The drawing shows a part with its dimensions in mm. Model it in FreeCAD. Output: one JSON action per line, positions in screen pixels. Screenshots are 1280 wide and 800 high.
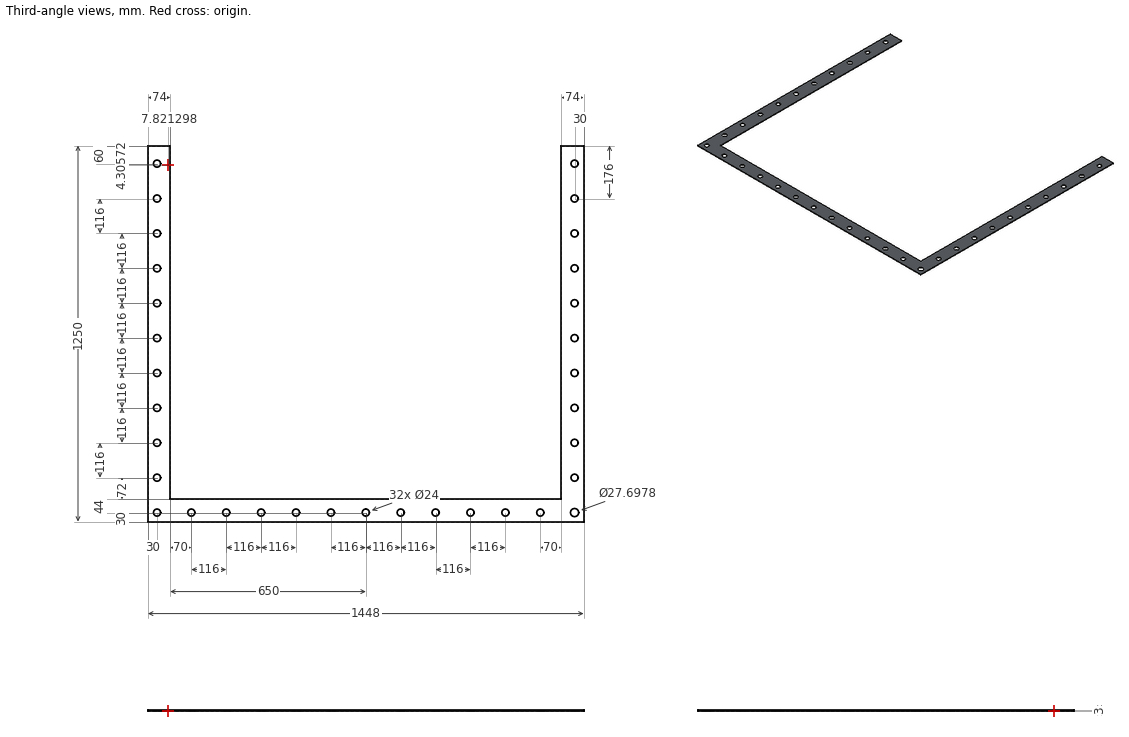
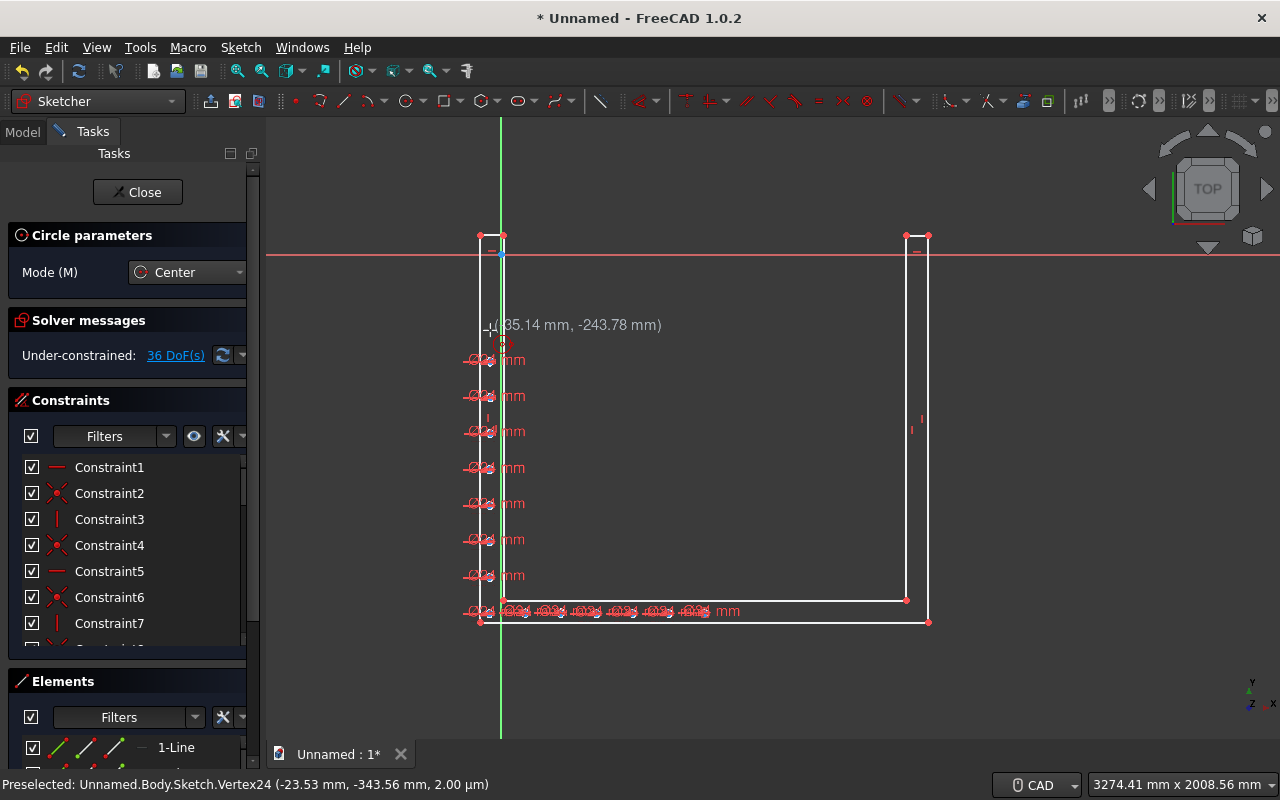
{"action": "scroll", "coordinate": [490, 325], "scroll_direction": "up", "scroll_amount": 3}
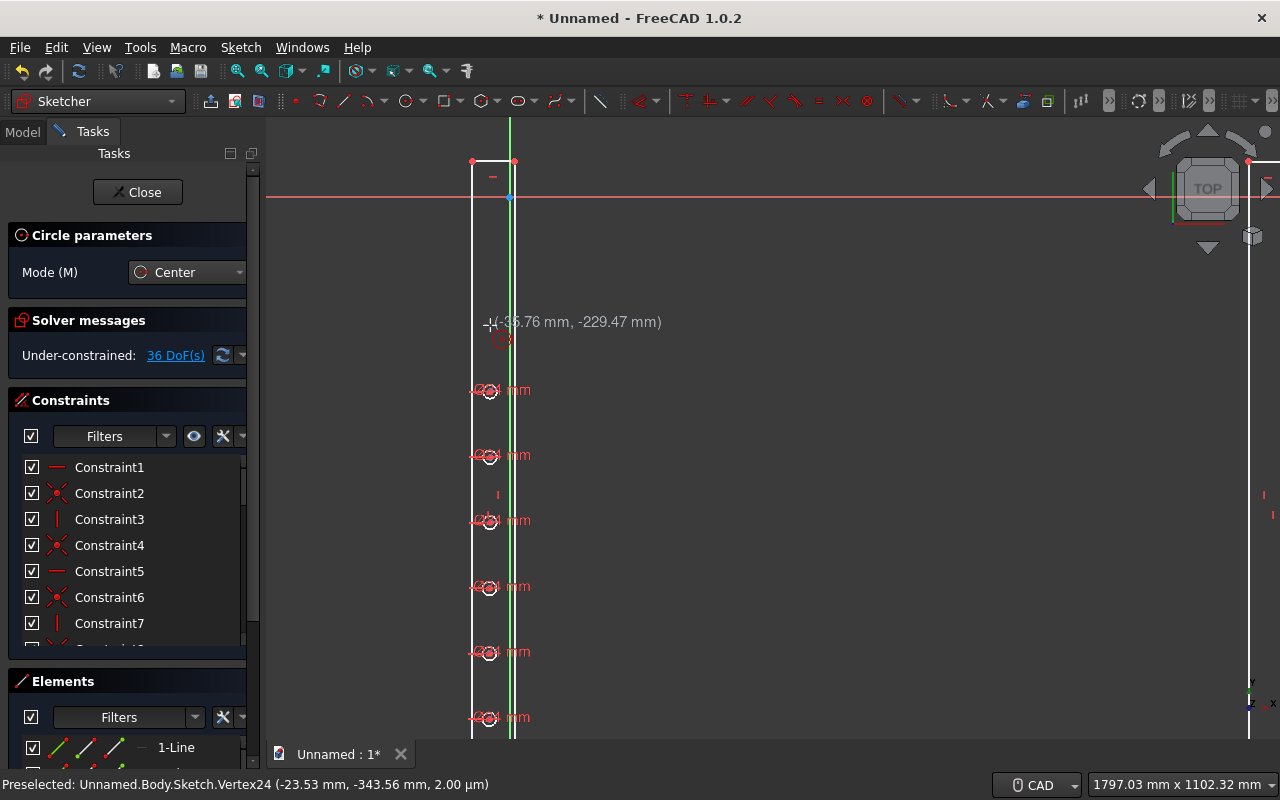
{"action": "left_click", "coordinate": [490, 326]}
{"action": "mouse_move", "coordinate": [494, 321]}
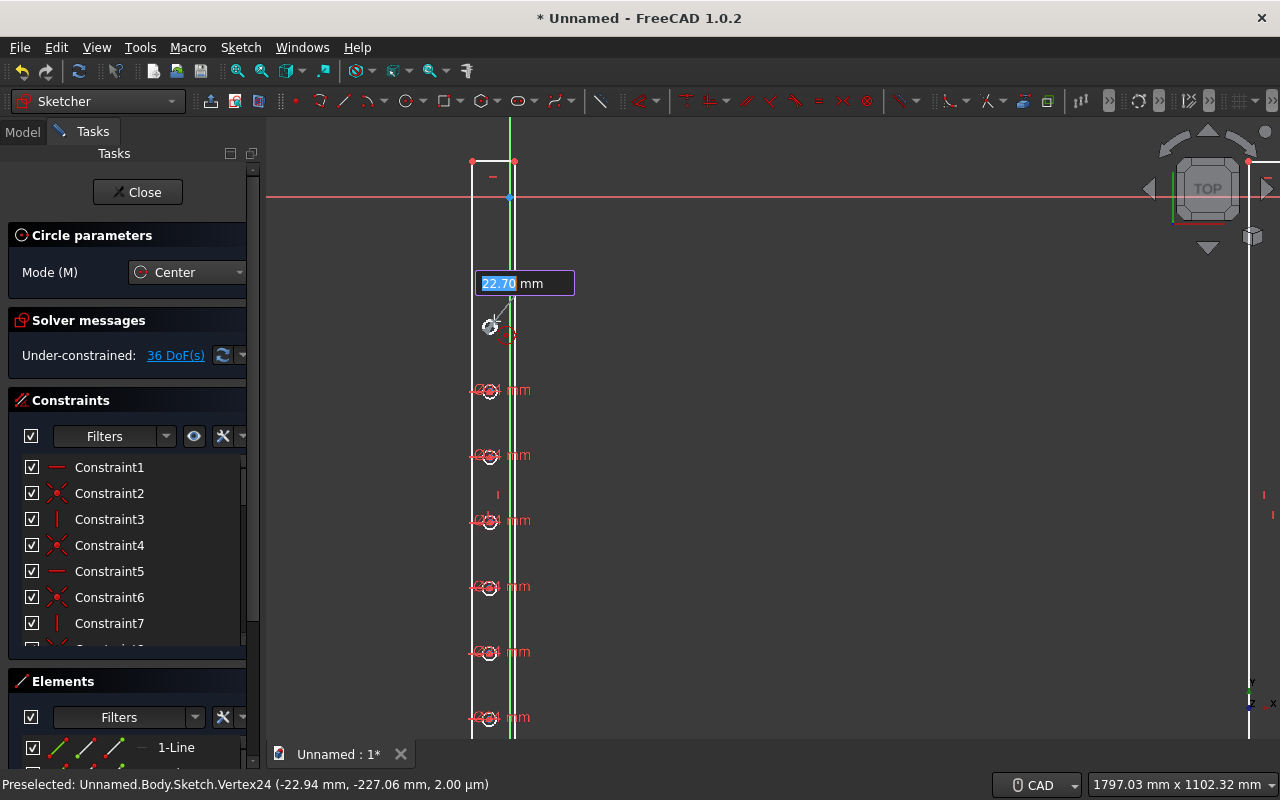
{"action": "type", "text": "24"}
{"action": "key", "text": "Return"}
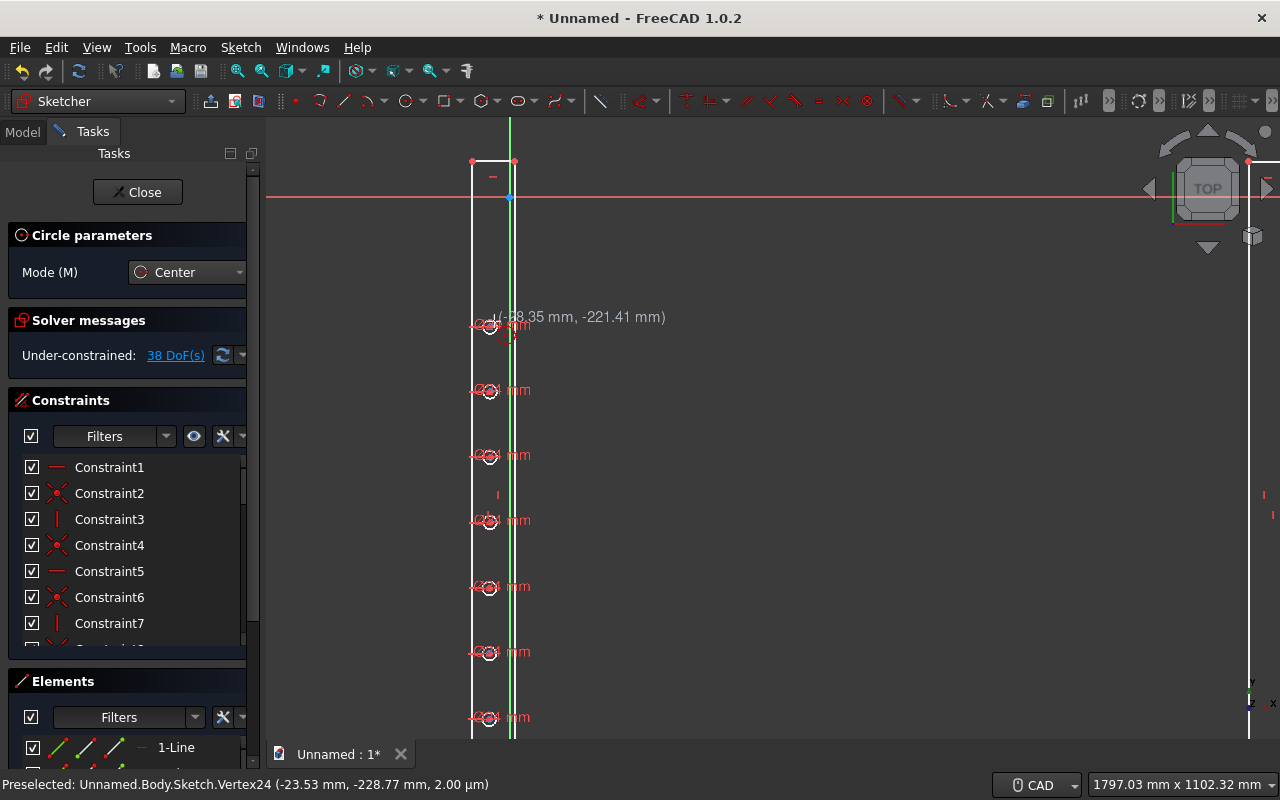
{"action": "scroll", "coordinate": [490, 260], "scroll_direction": "up", "scroll_amount": 7}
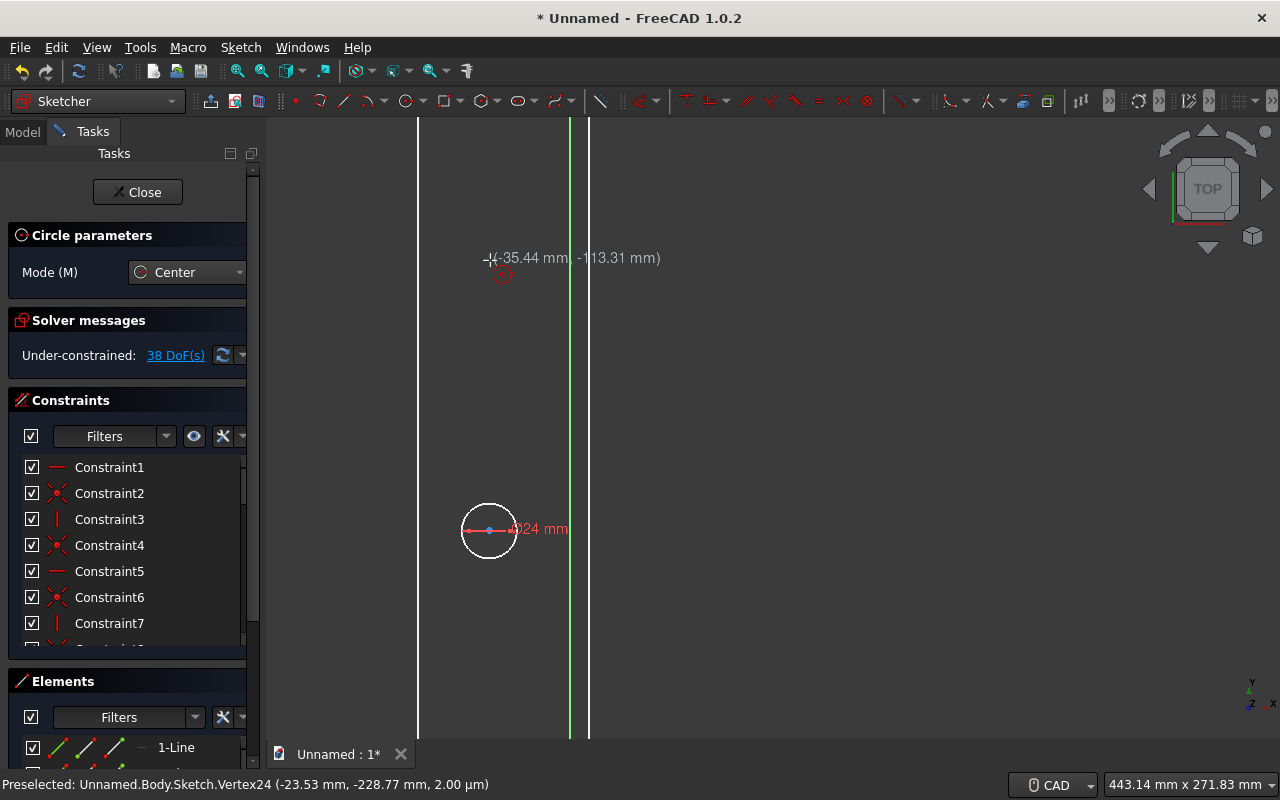
{"action": "scroll", "coordinate": [490, 294], "scroll_direction": "down", "scroll_amount": 10}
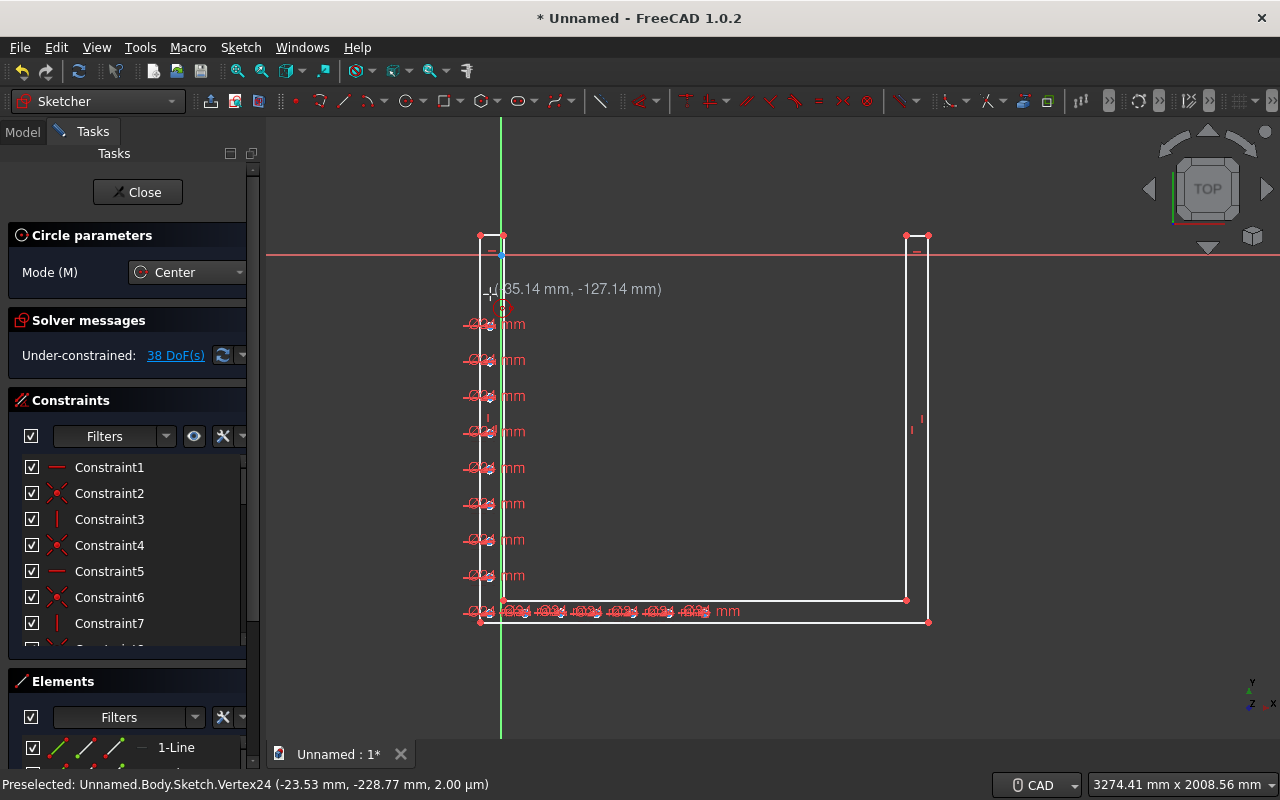
{"action": "scroll", "coordinate": [490, 290], "scroll_direction": "up", "scroll_amount": 3}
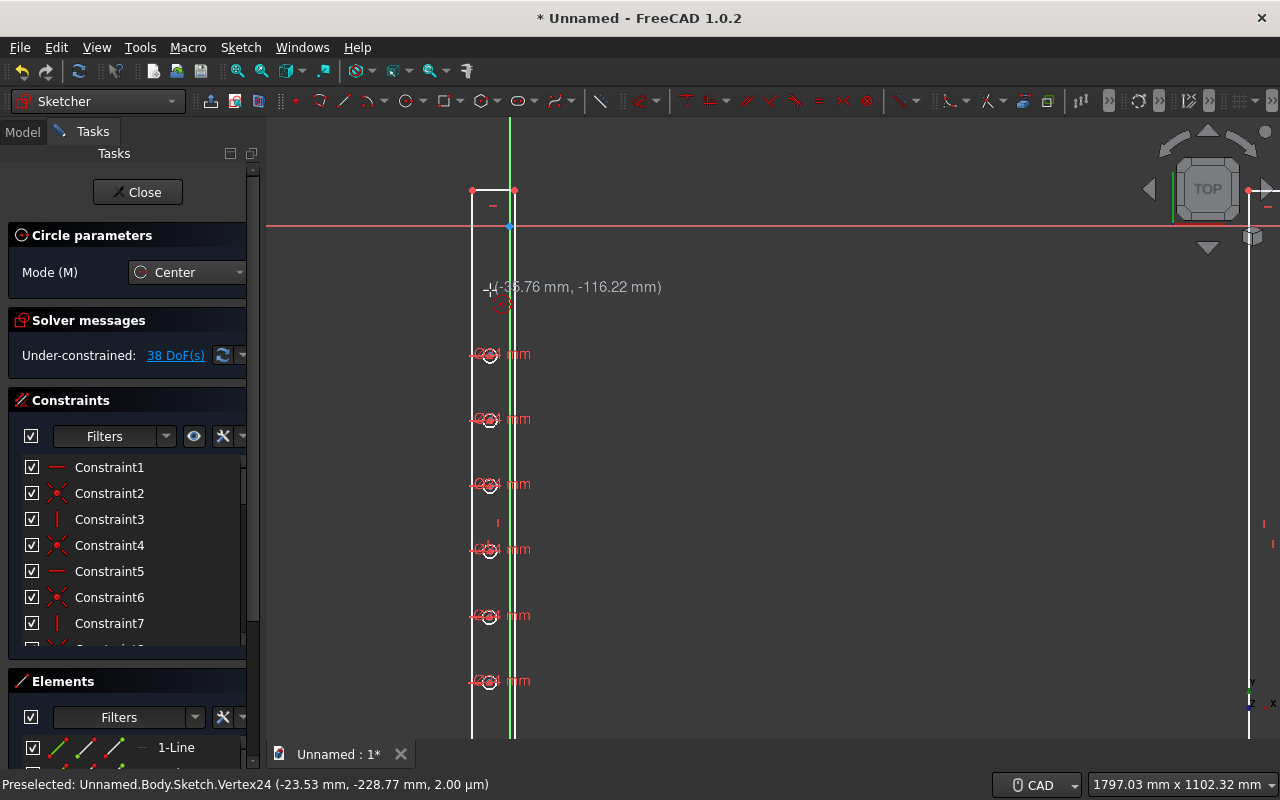
{"action": "left_click", "coordinate": [490, 289]}
{"action": "mouse_move", "coordinate": [494, 284]}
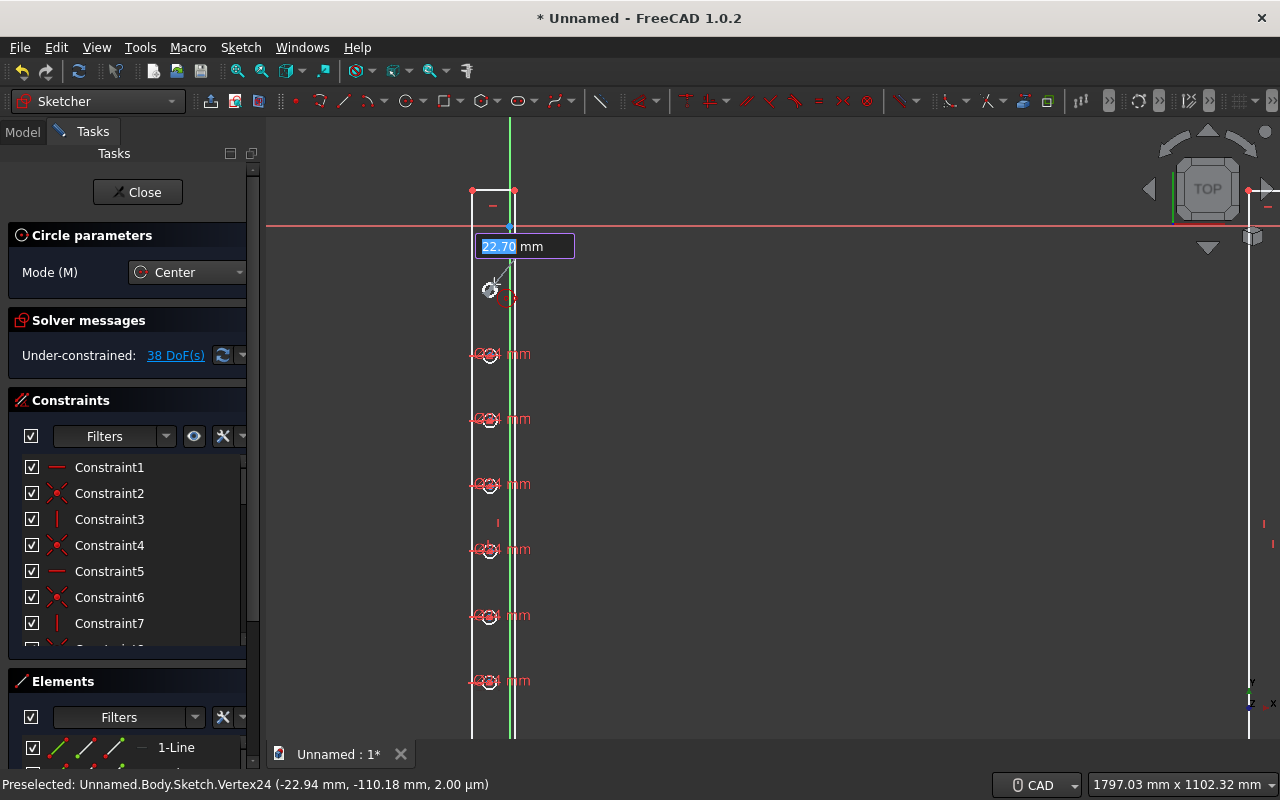
{"action": "type", "text": "24"}
{"action": "key", "text": "Return"}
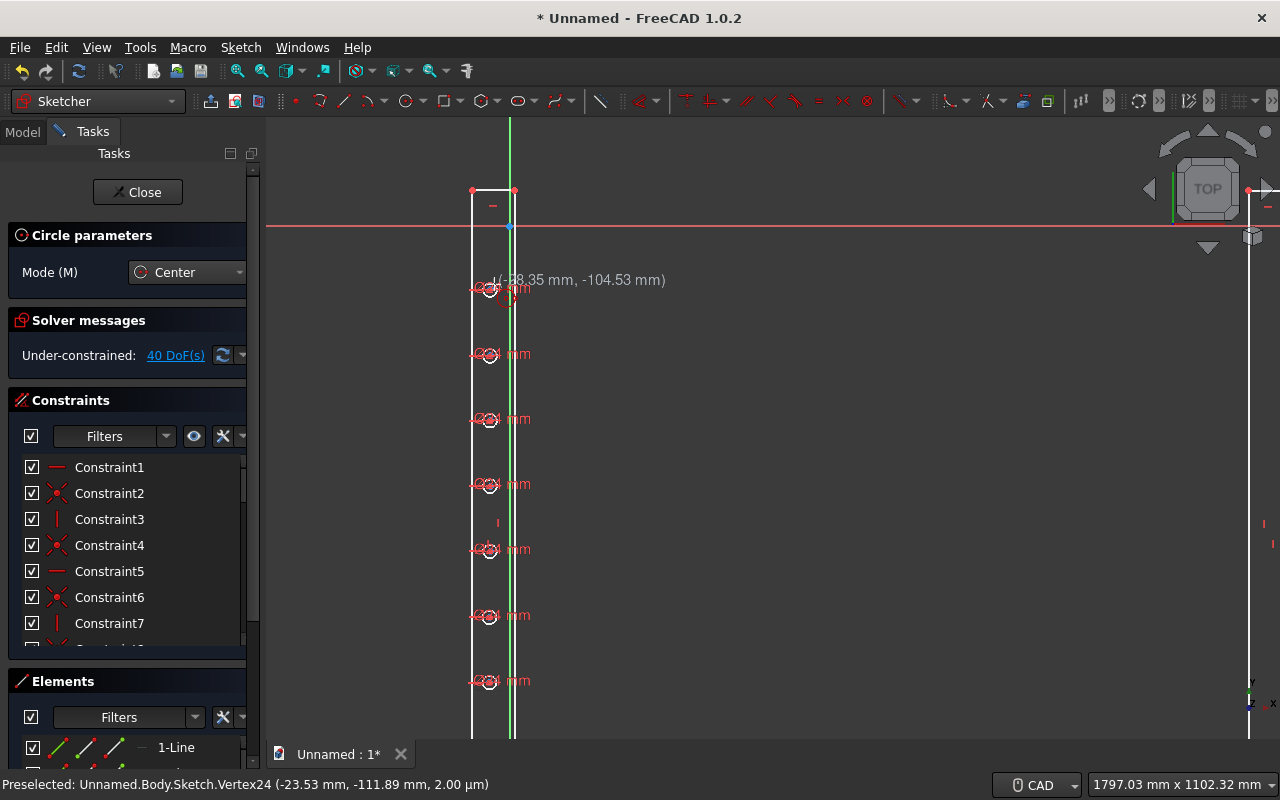
{"action": "scroll", "coordinate": [490, 224], "scroll_direction": "up", "scroll_amount": 10}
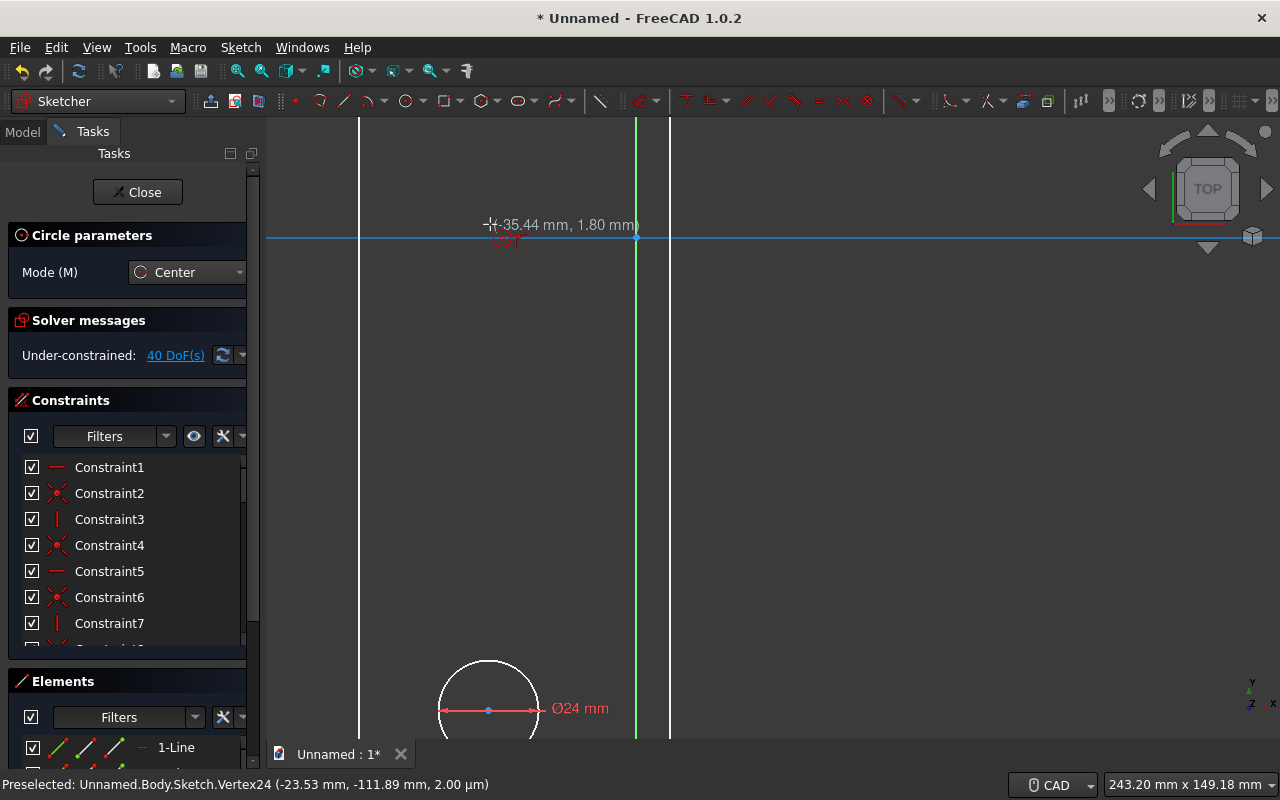
{"action": "left_click", "coordinate": [485, 220]}